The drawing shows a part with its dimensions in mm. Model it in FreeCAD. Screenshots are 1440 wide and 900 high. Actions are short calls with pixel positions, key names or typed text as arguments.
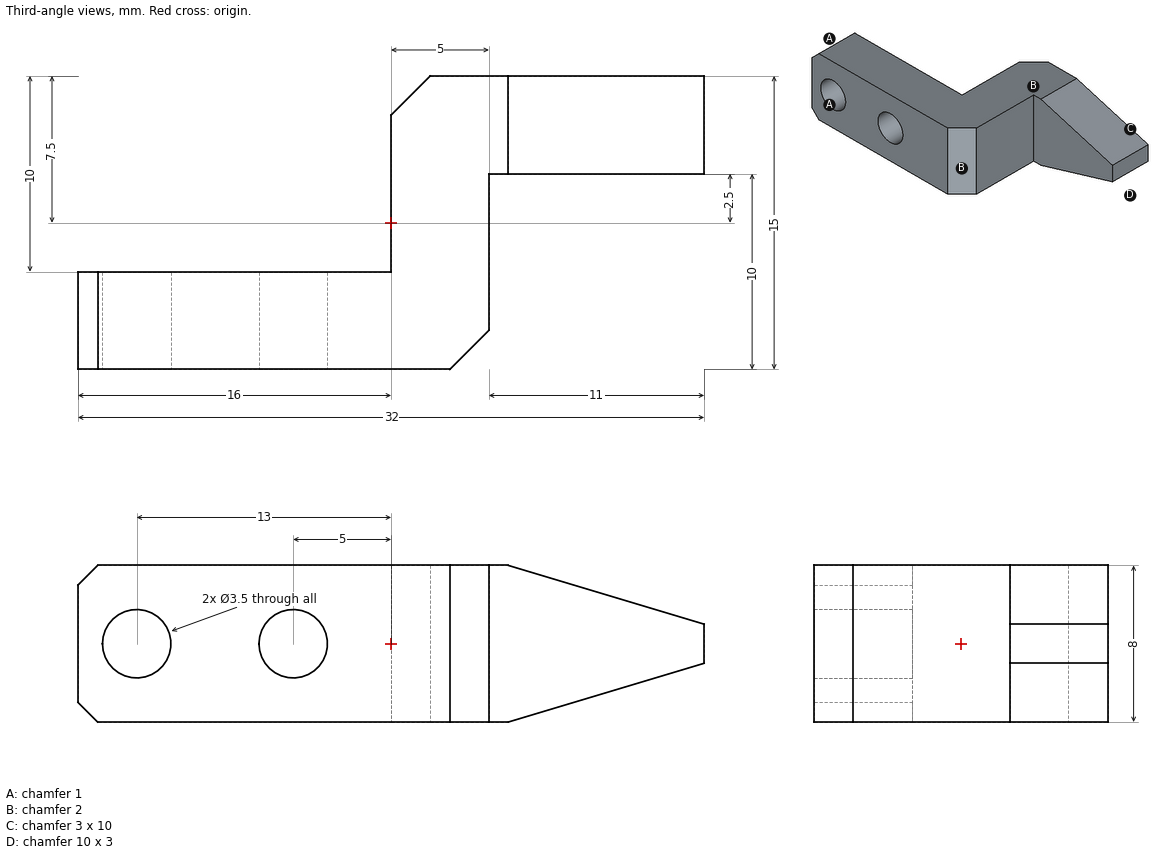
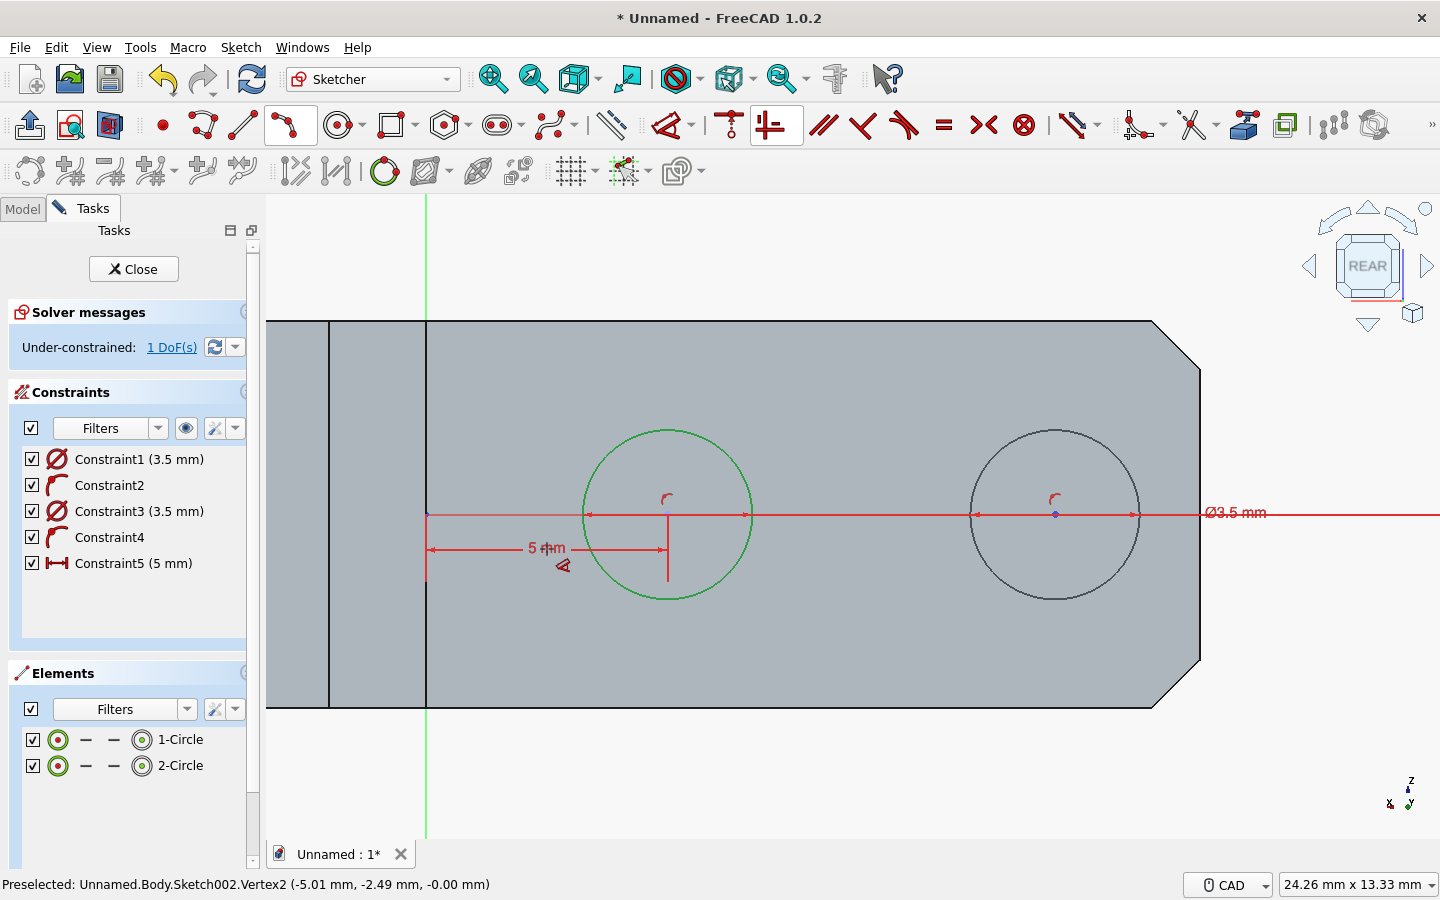
click(1055, 515)
click(885, 549)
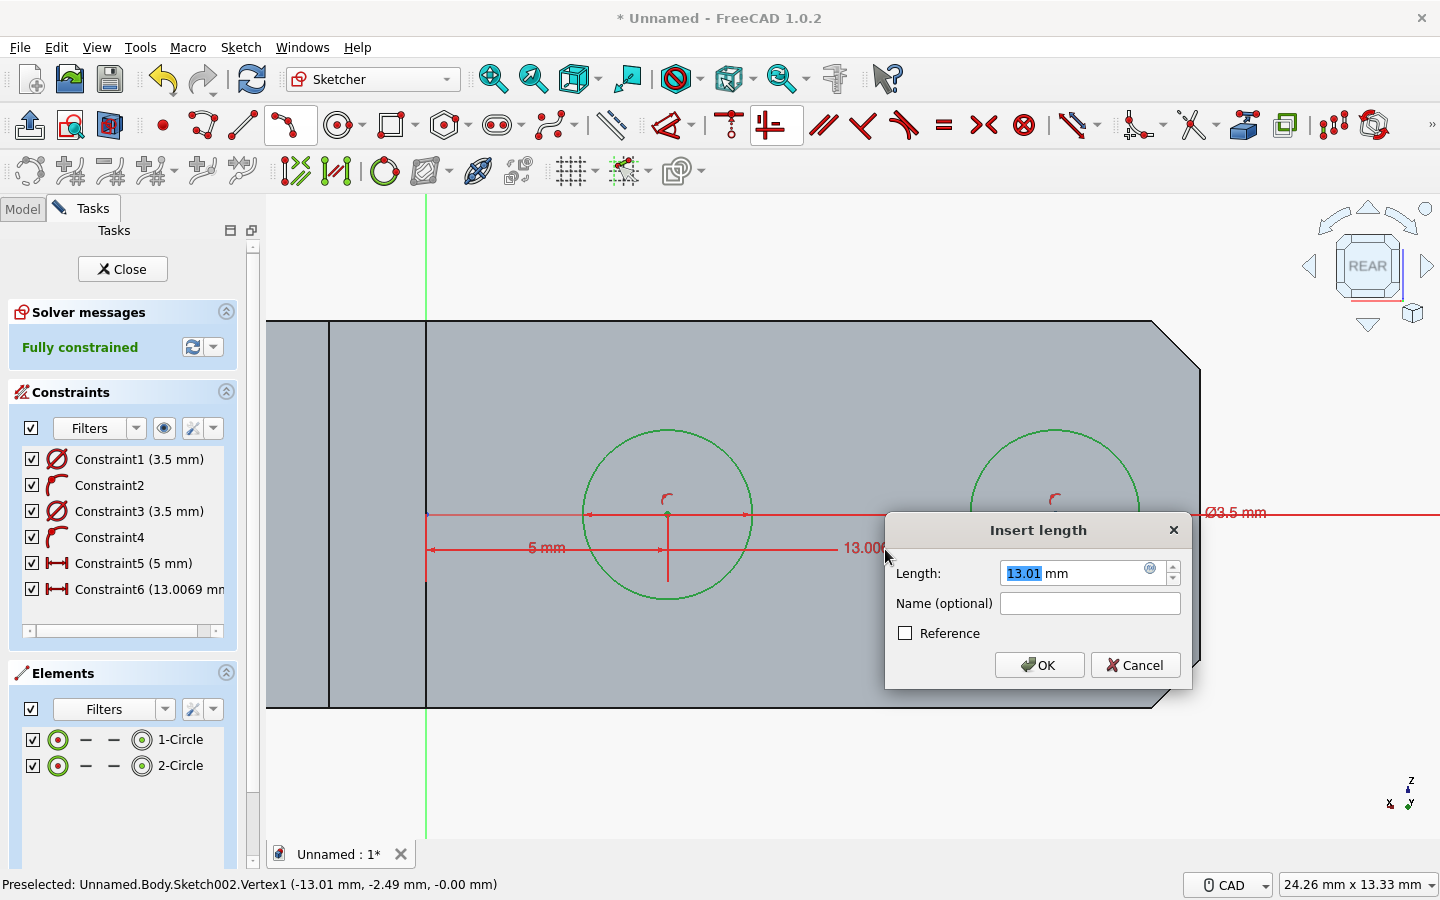
text(13)
key(Return)
key(Escape)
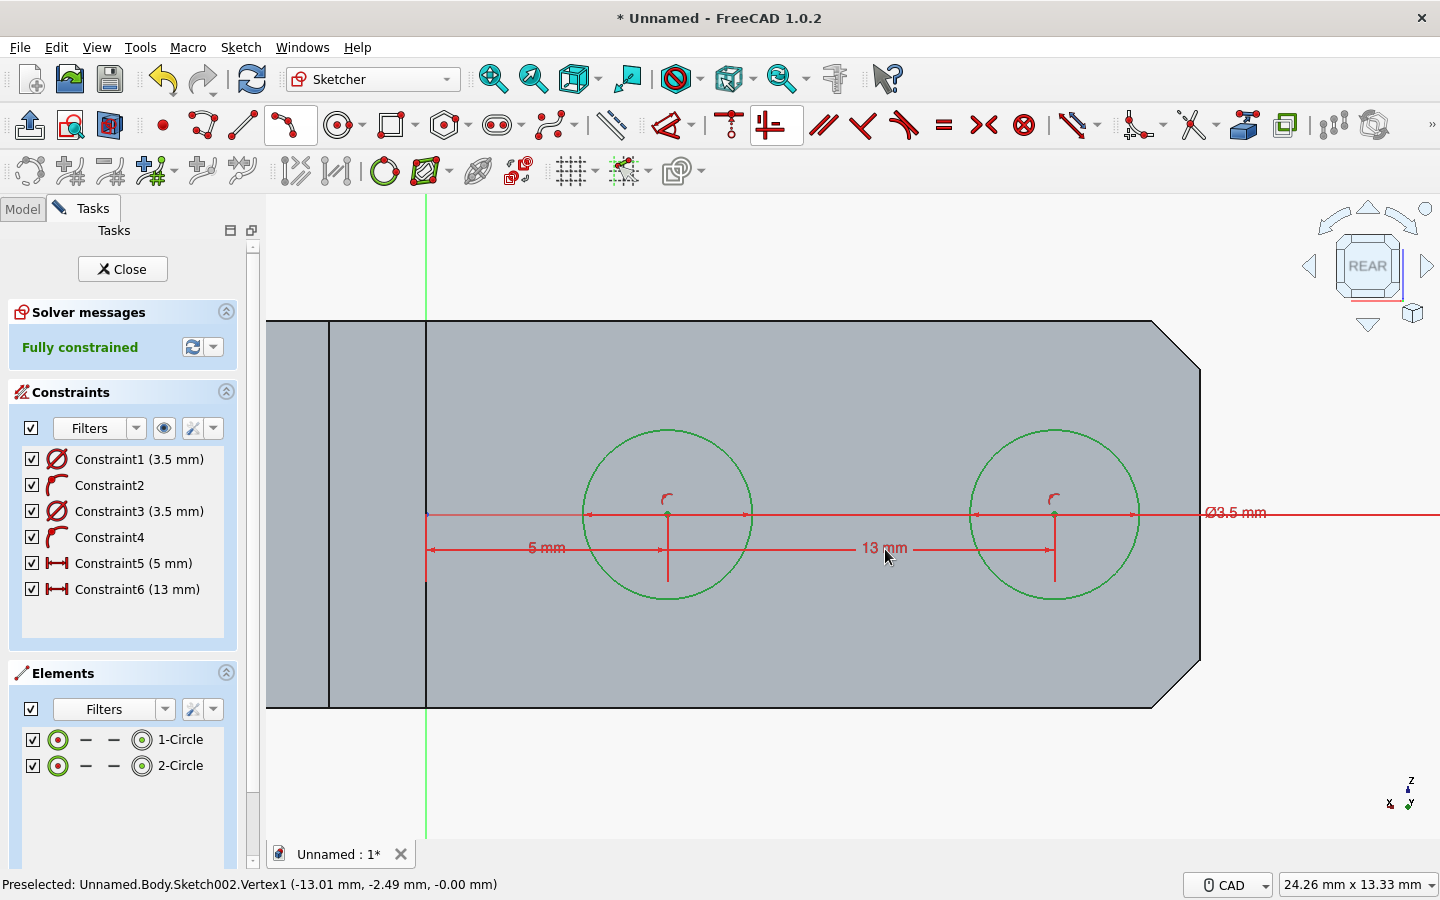
click(123, 269)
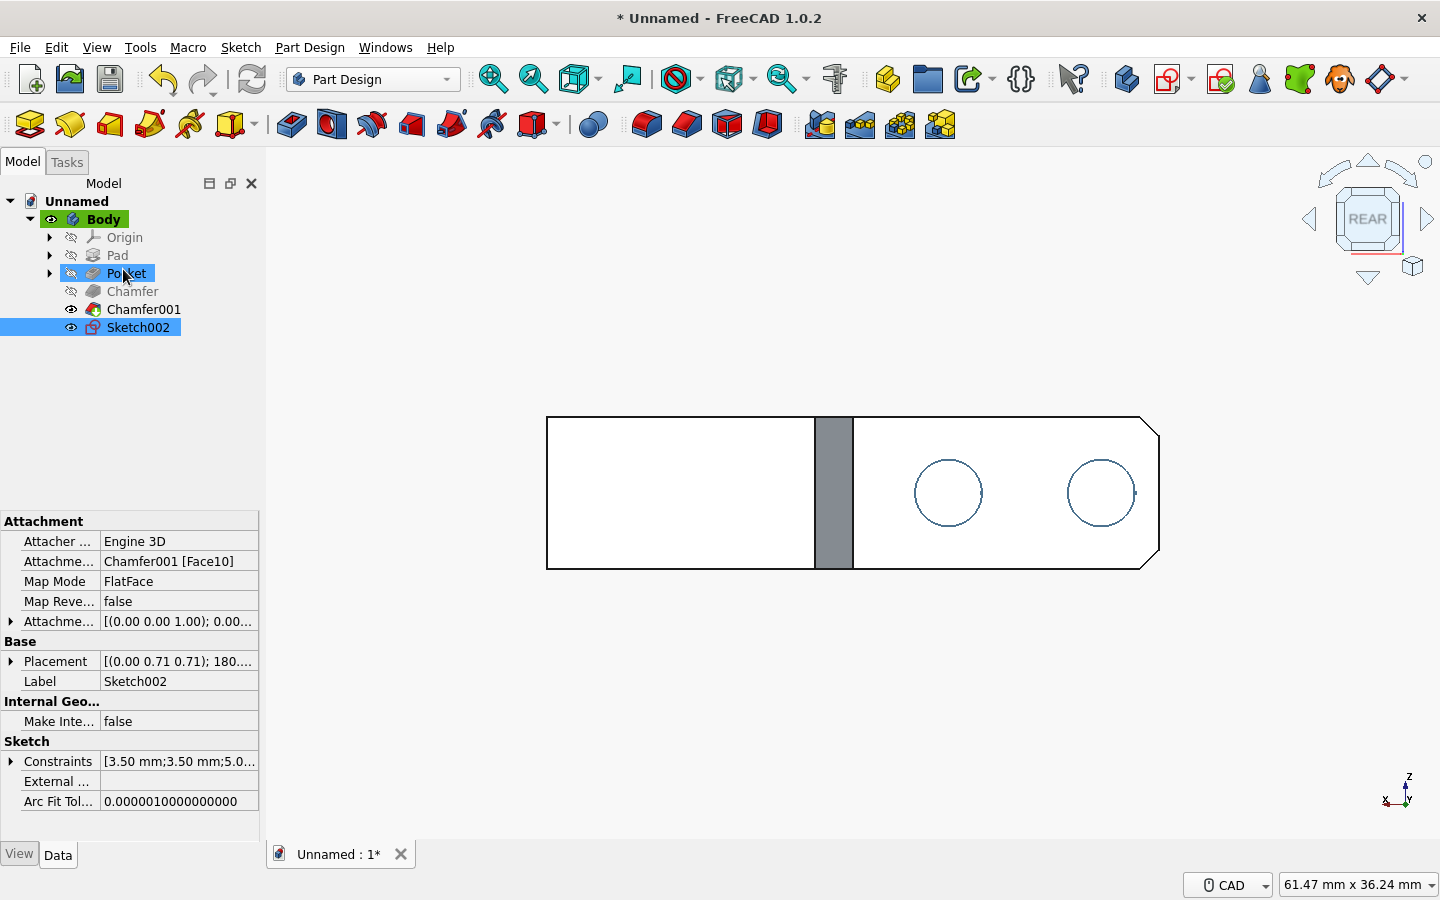
click(332, 124)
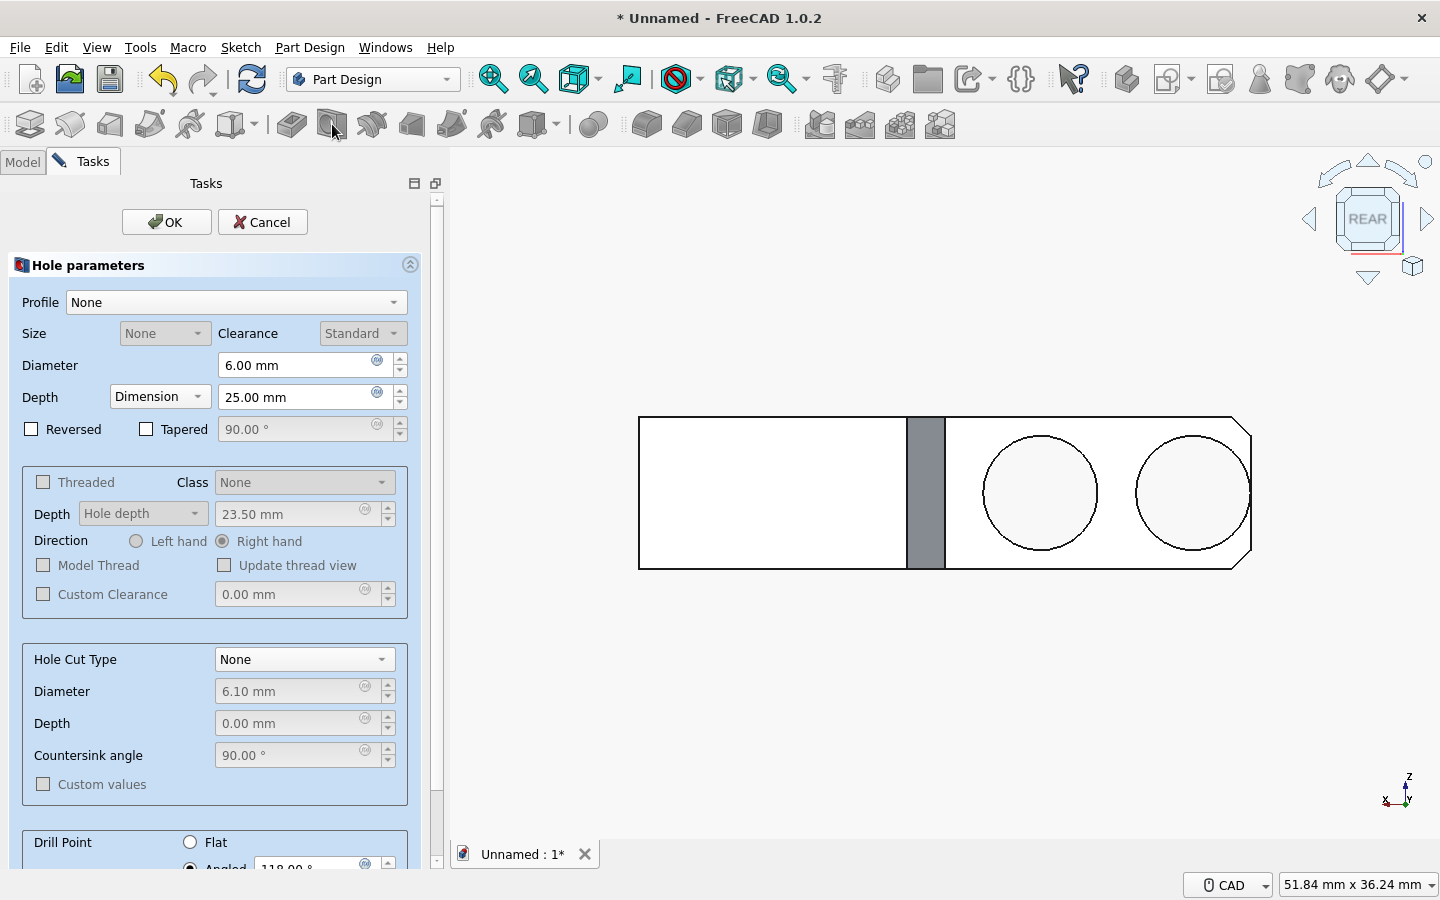
triple_click(305, 365)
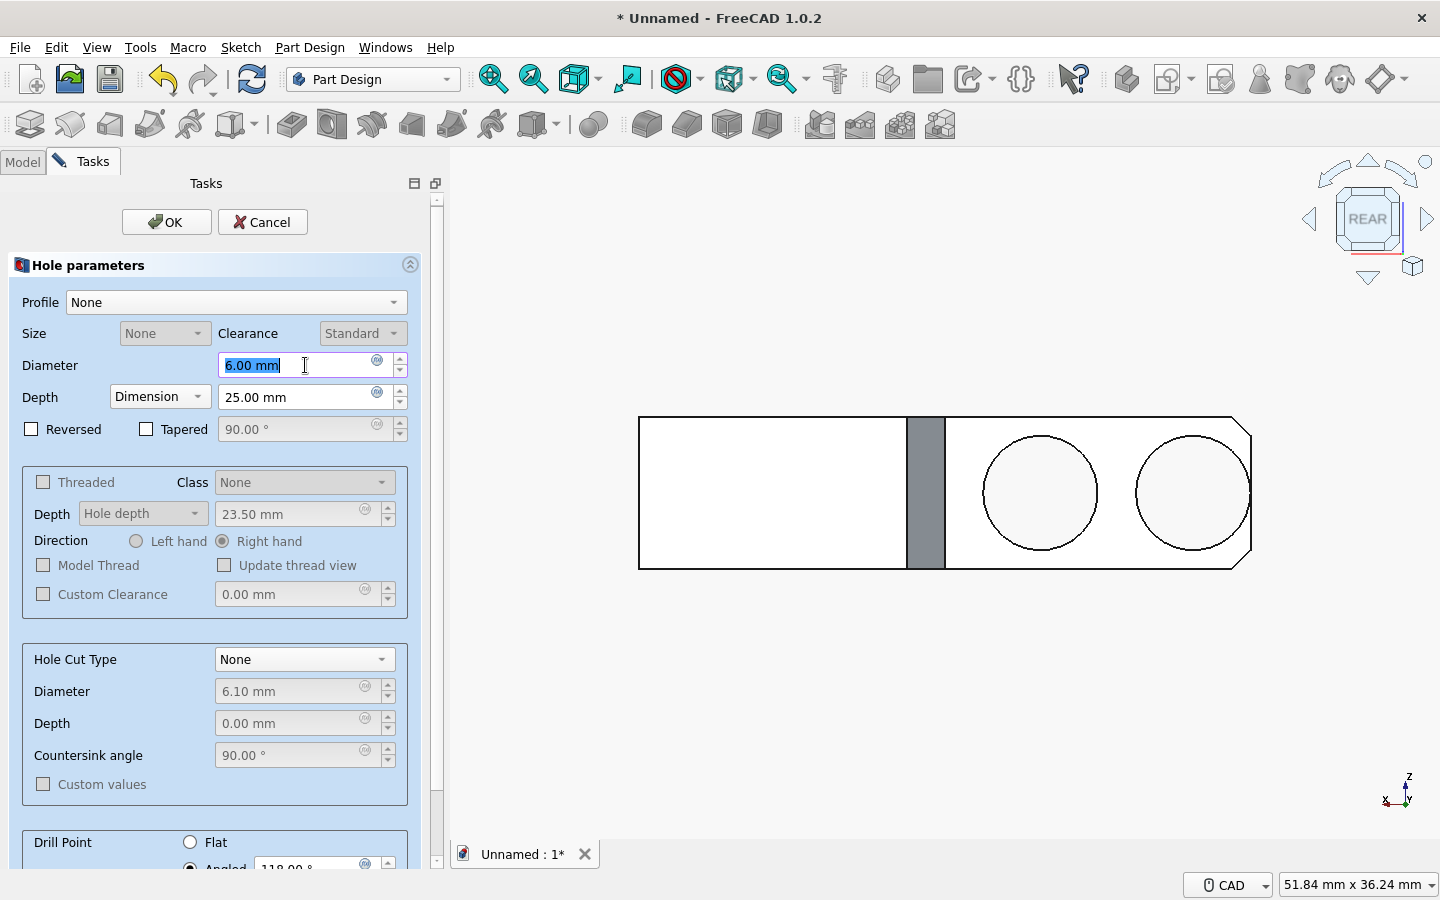
text(3.5)
key(Tab)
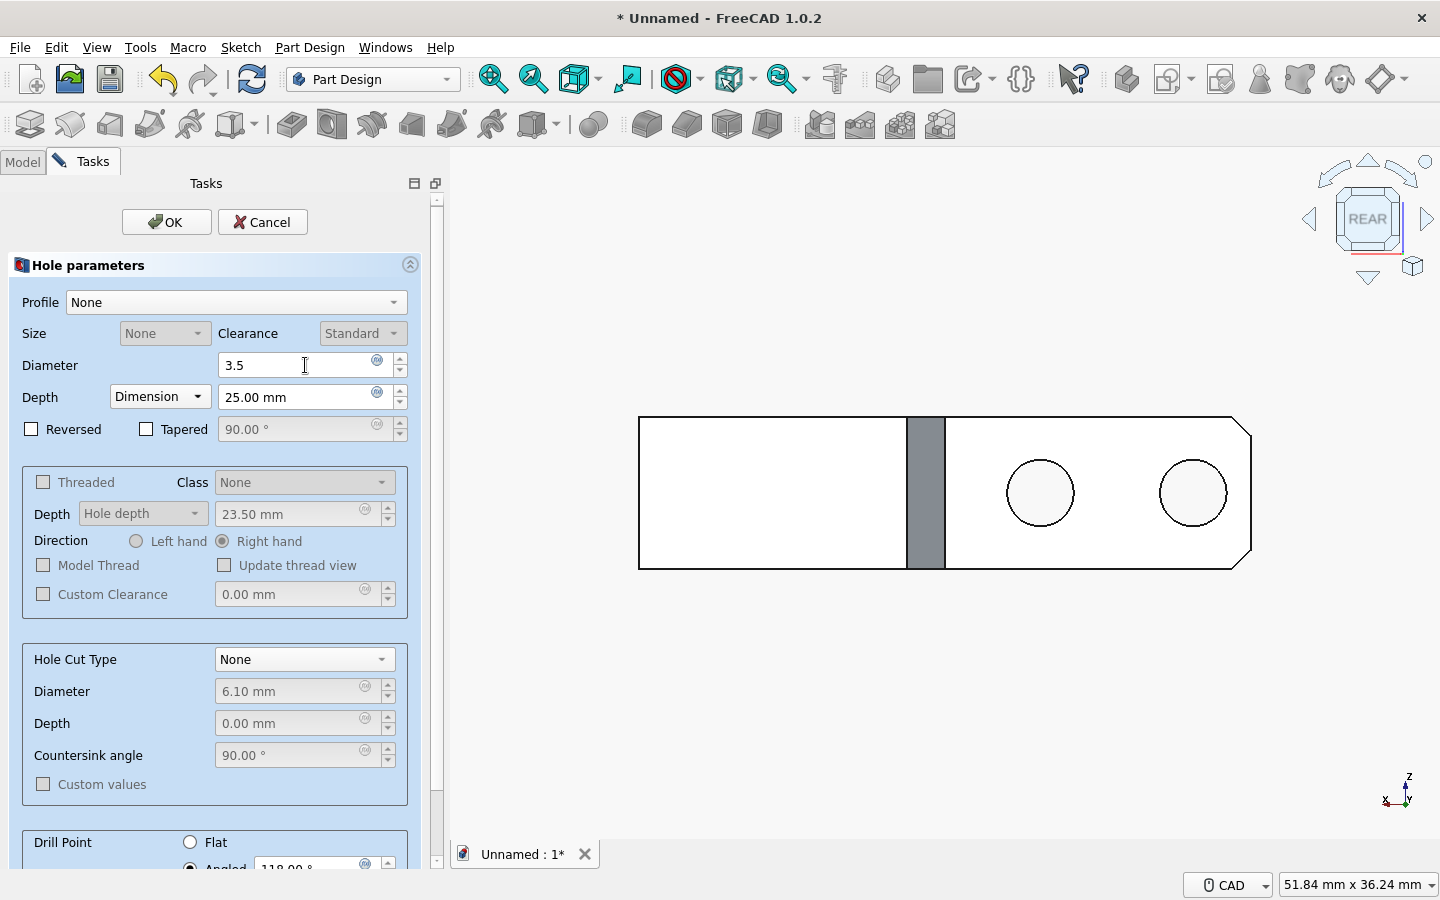
click(161, 396)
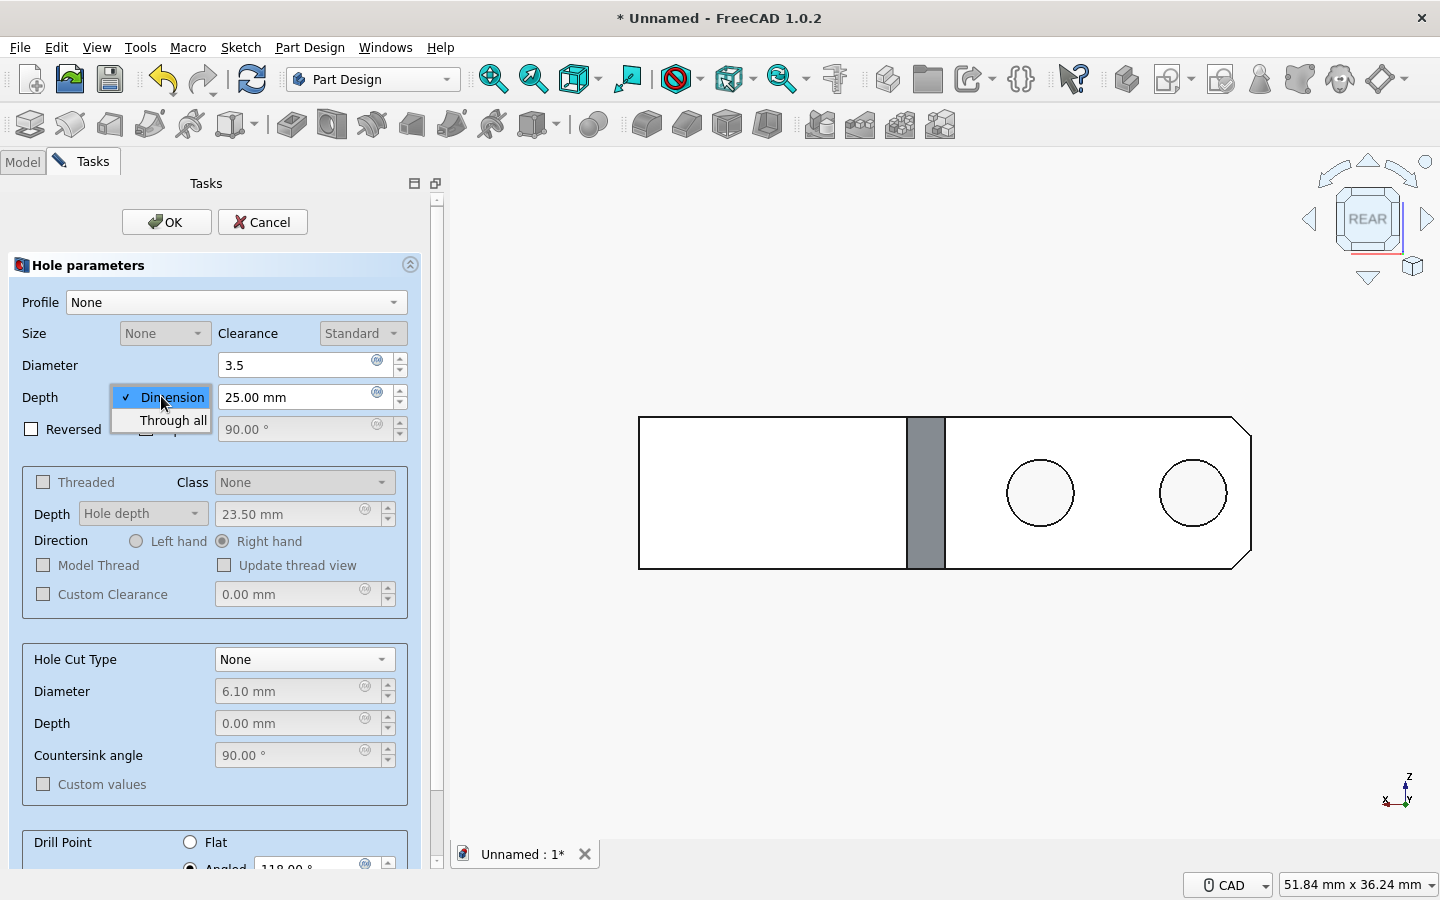
click(160, 420)